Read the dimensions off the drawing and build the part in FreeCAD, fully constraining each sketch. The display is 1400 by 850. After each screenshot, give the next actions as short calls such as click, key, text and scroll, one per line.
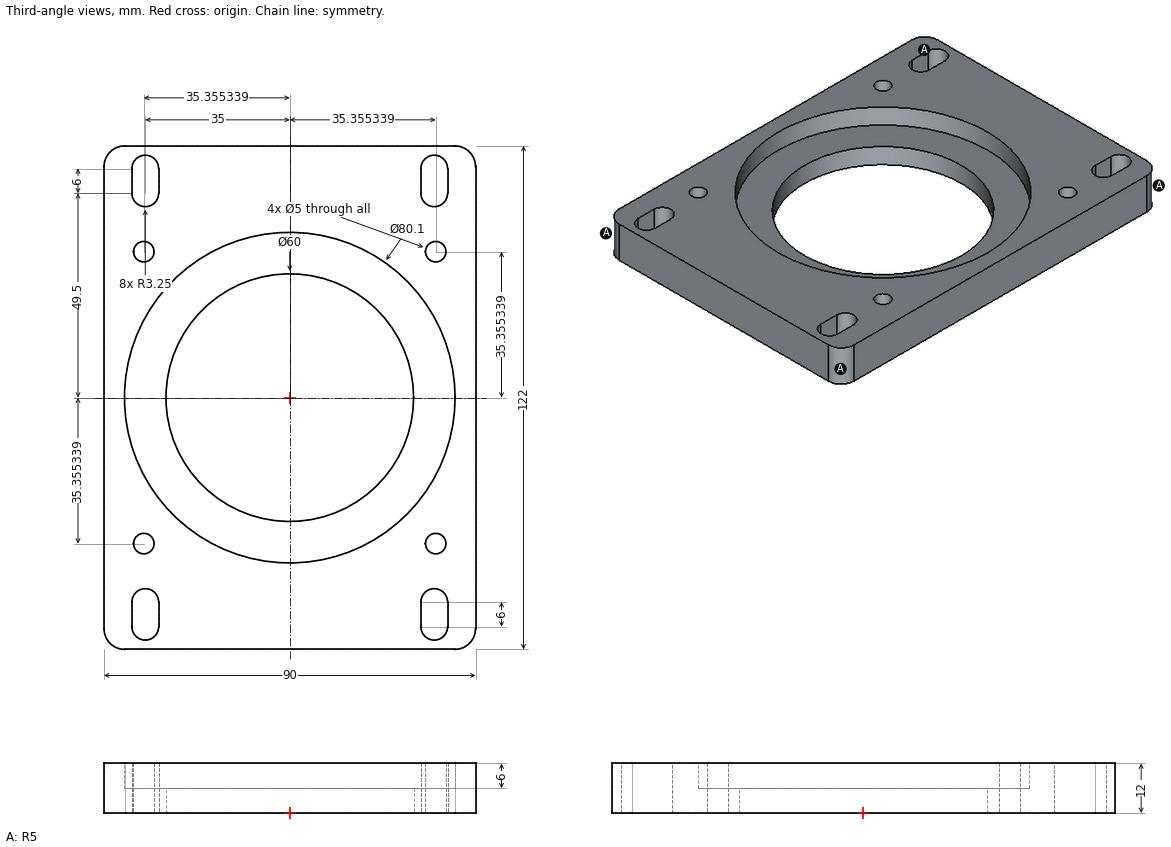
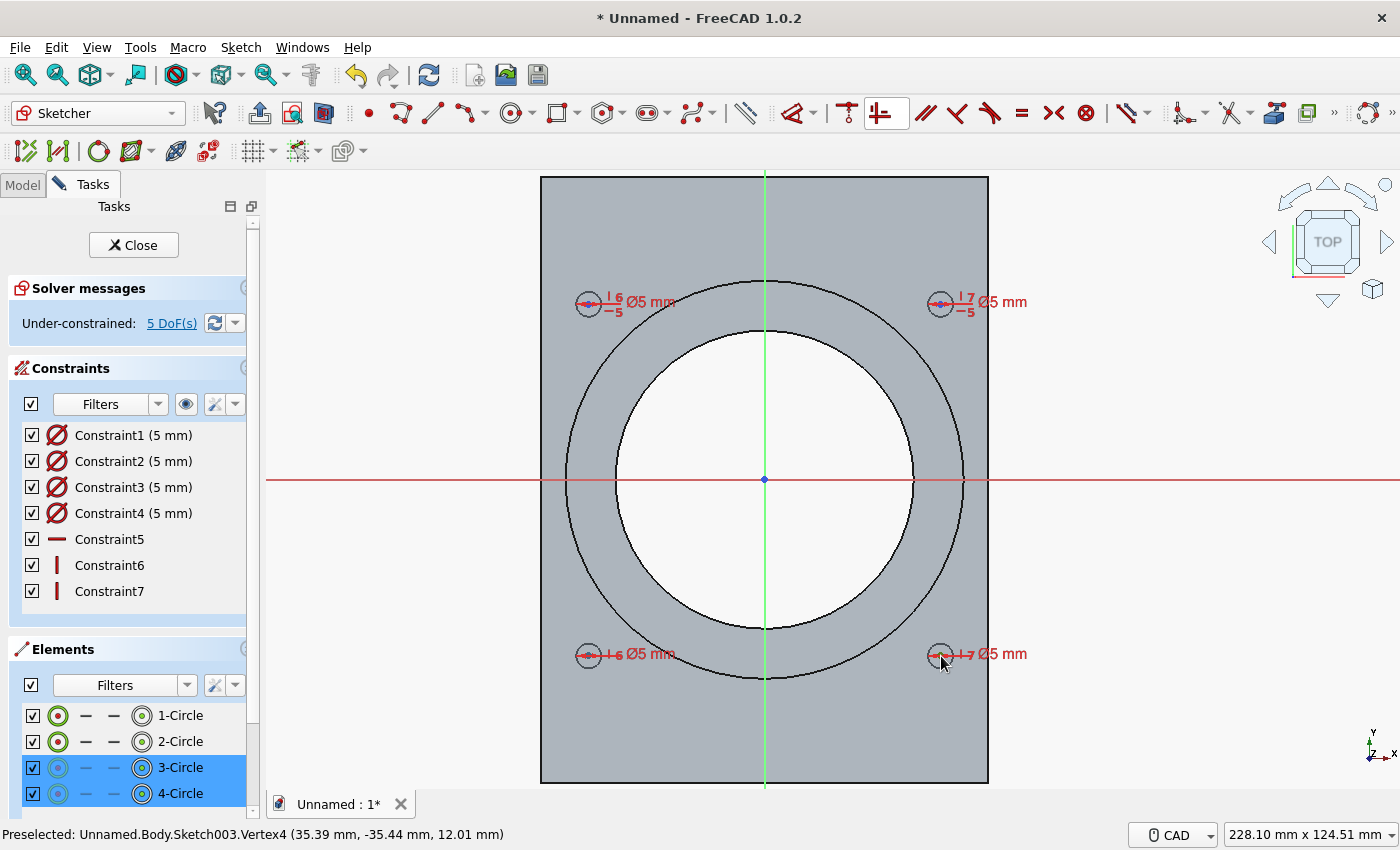
click(904, 114)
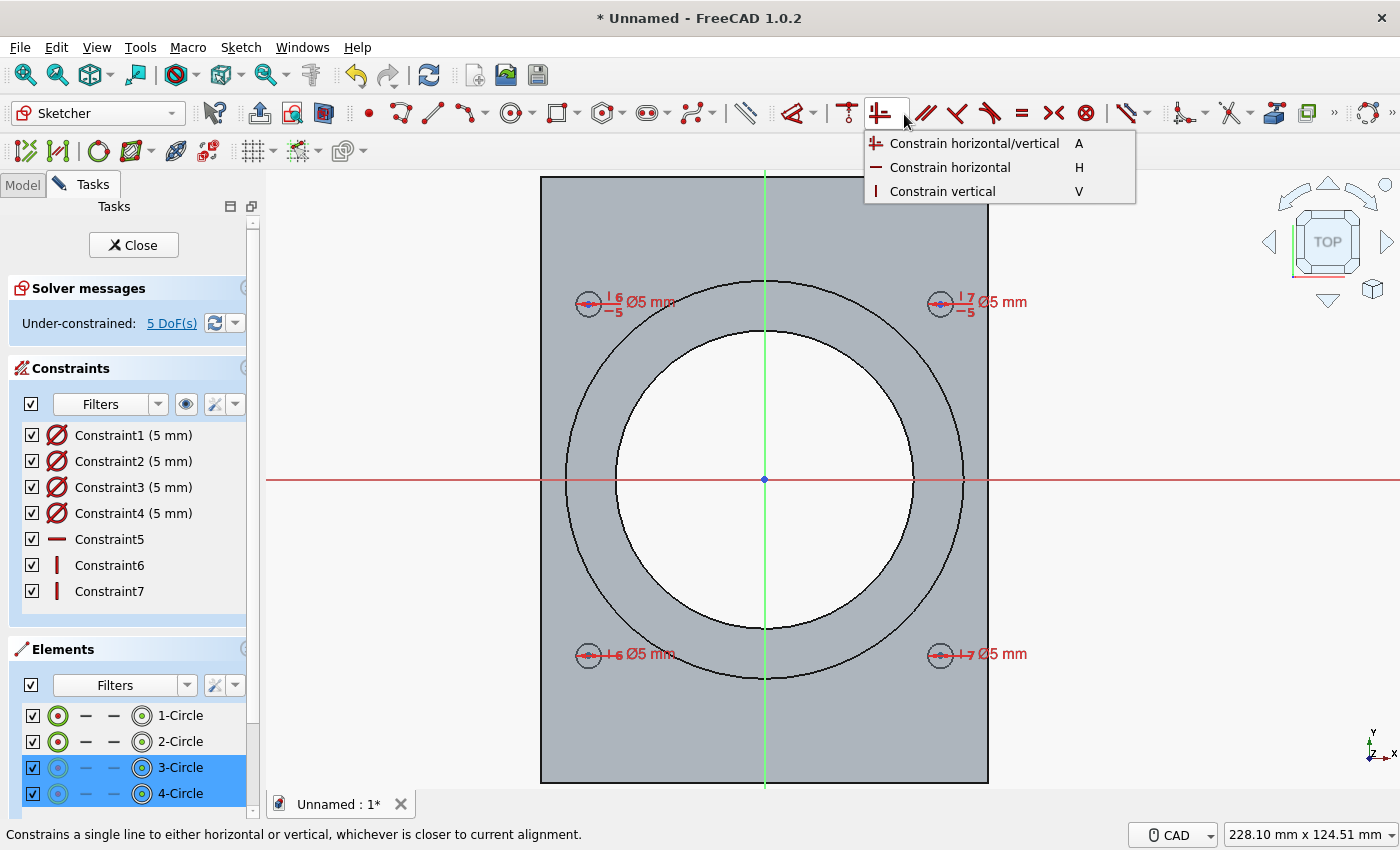
click(1000, 167)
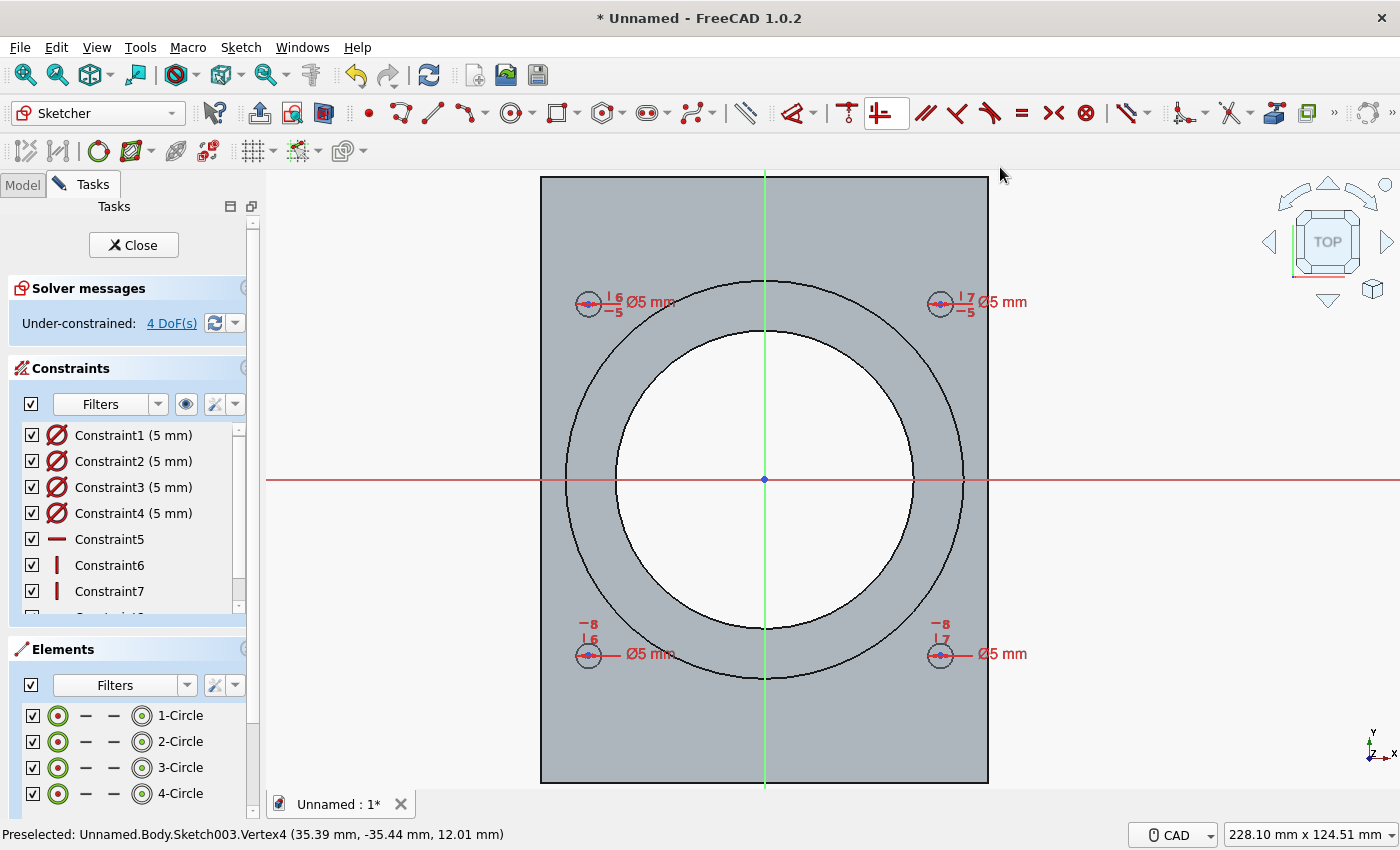
click(941, 304)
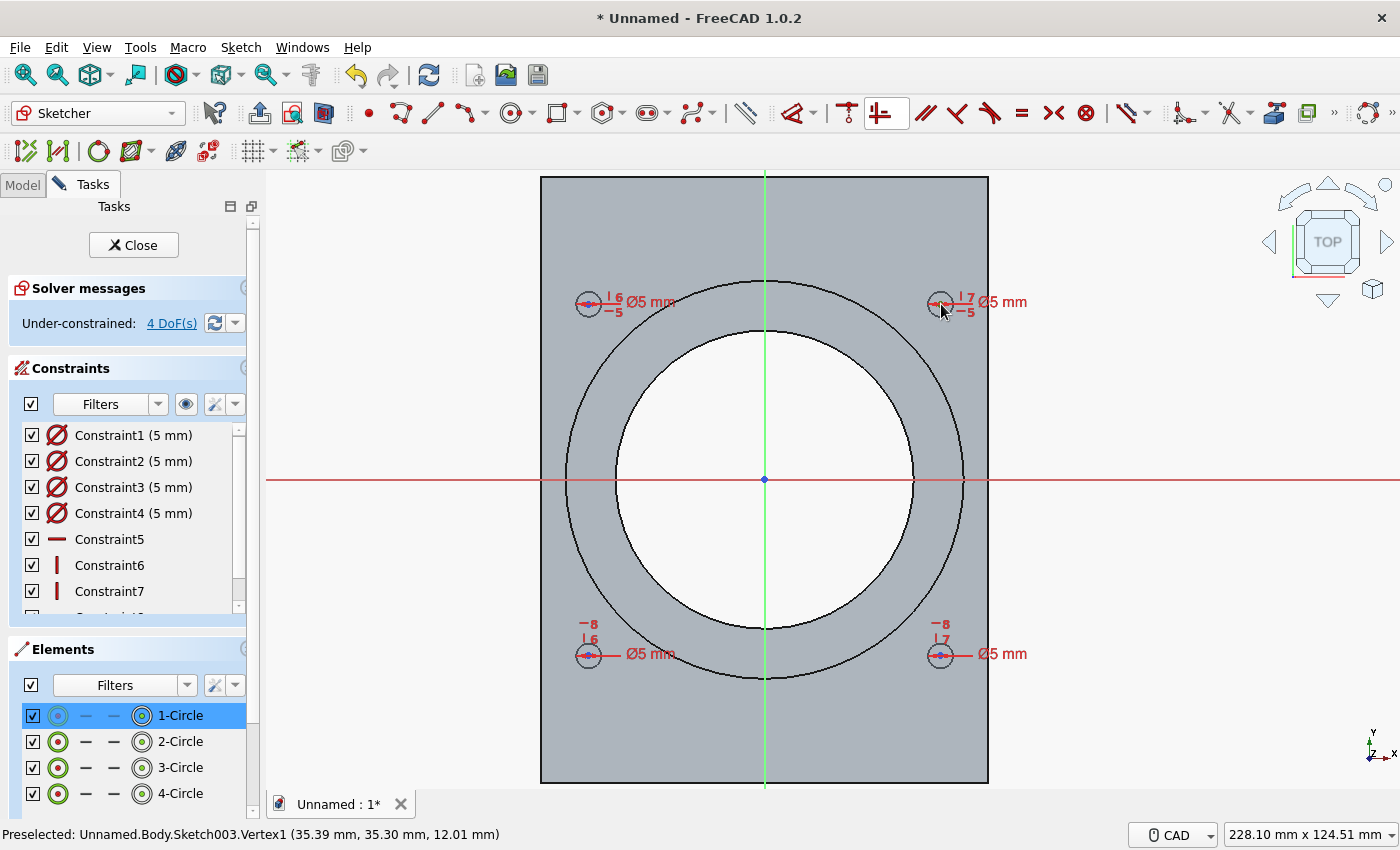
click(816, 114)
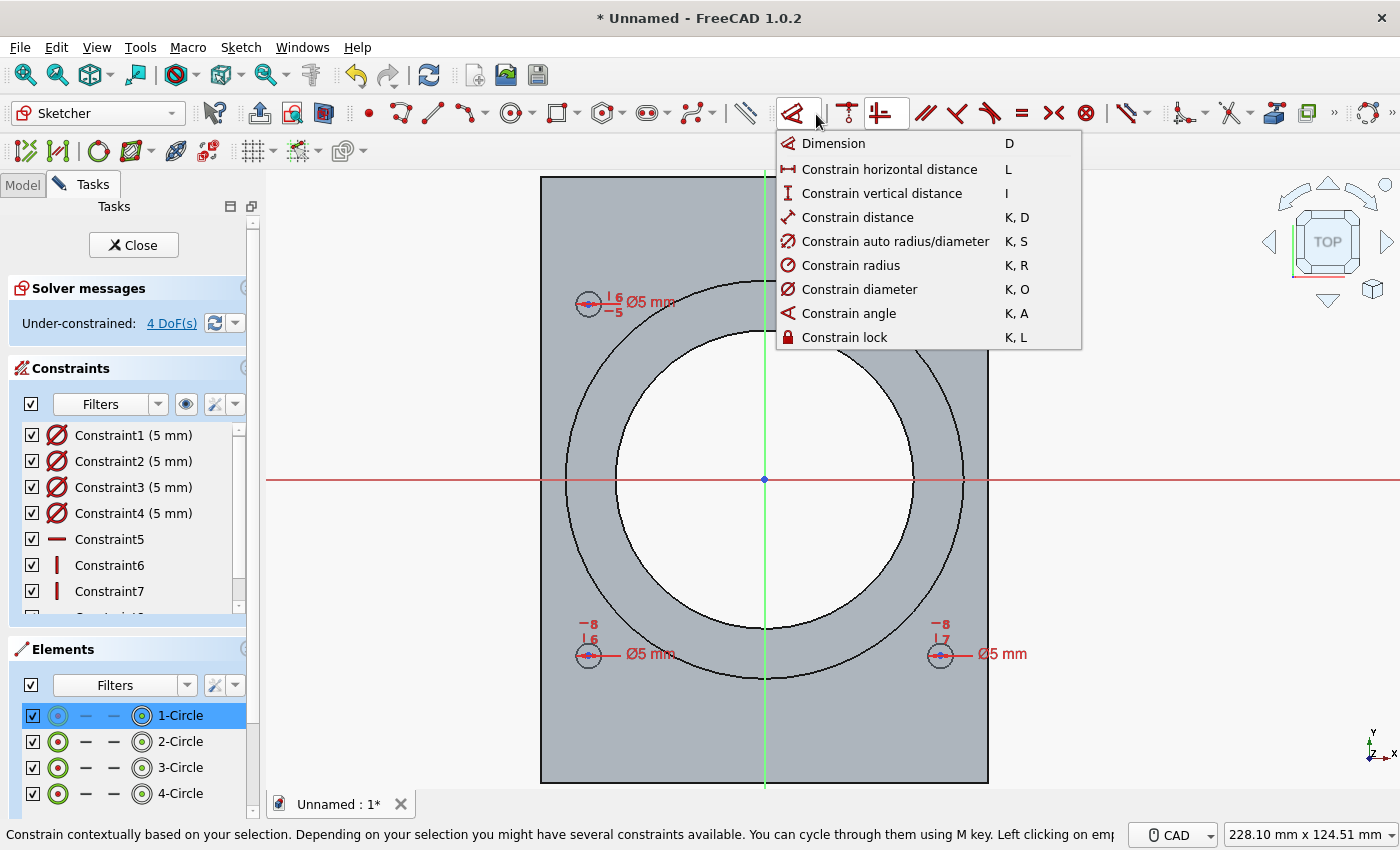
click(929, 169)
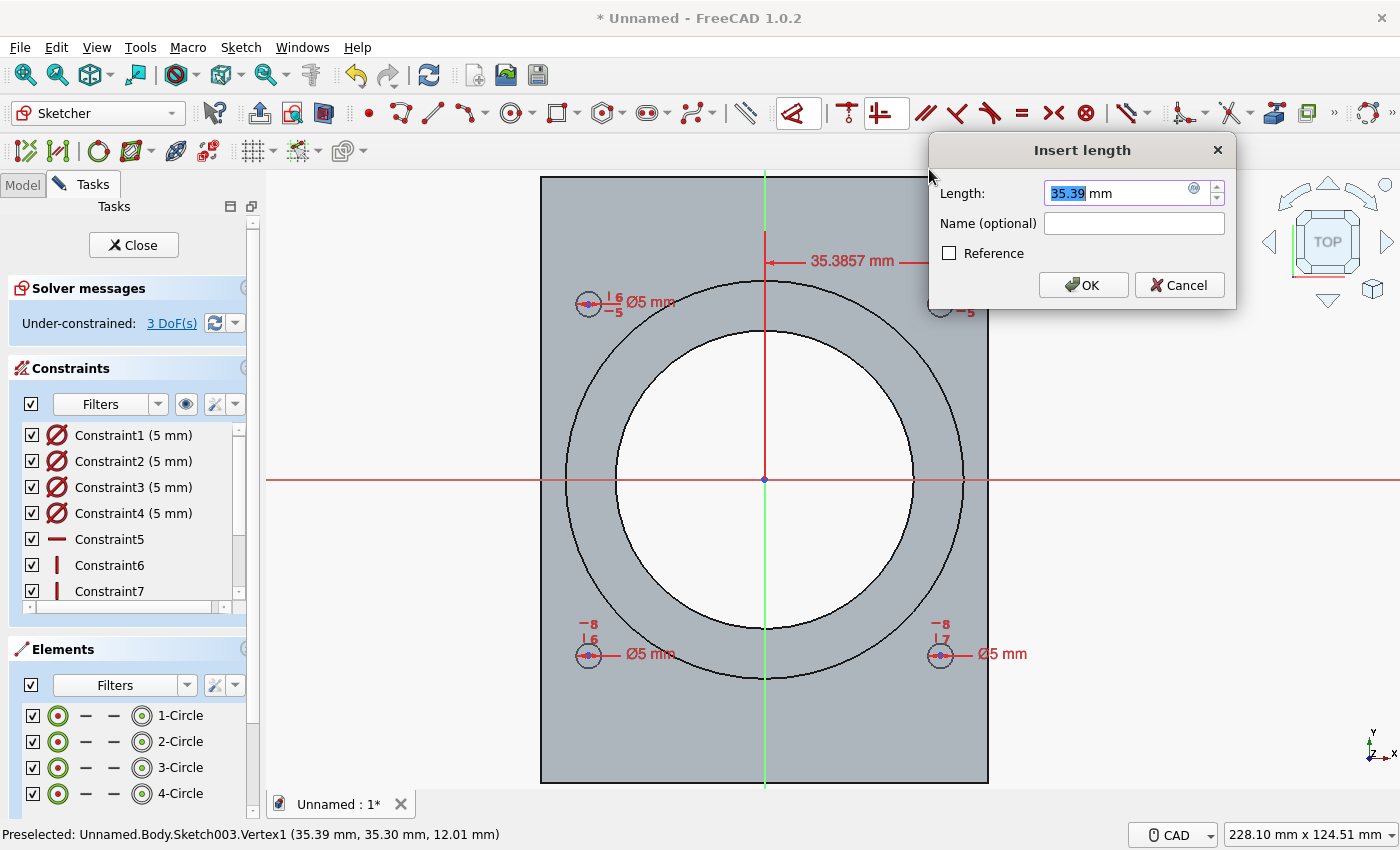
text(35.355339)
key(Return)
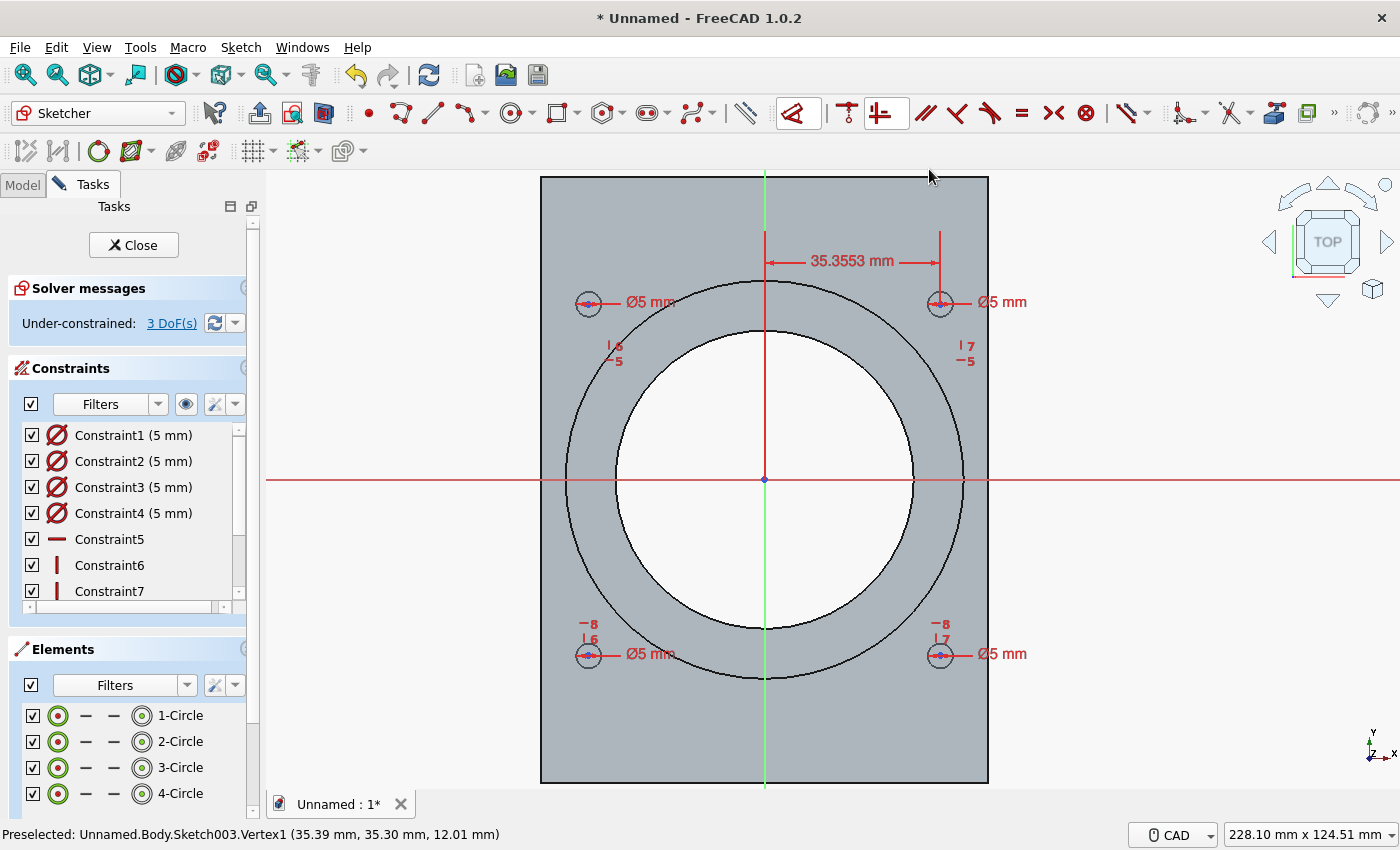
click(940, 304)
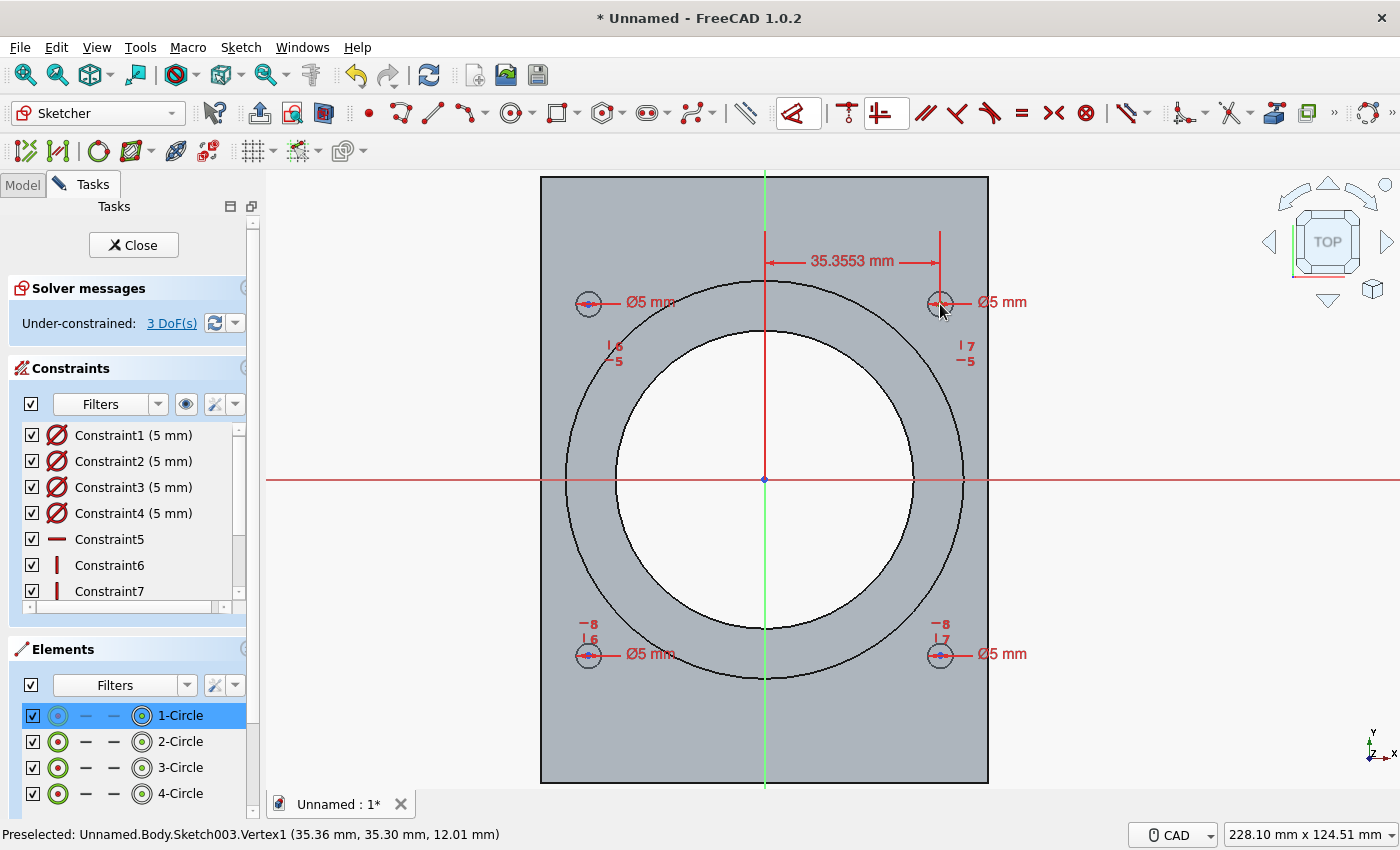
click(816, 114)